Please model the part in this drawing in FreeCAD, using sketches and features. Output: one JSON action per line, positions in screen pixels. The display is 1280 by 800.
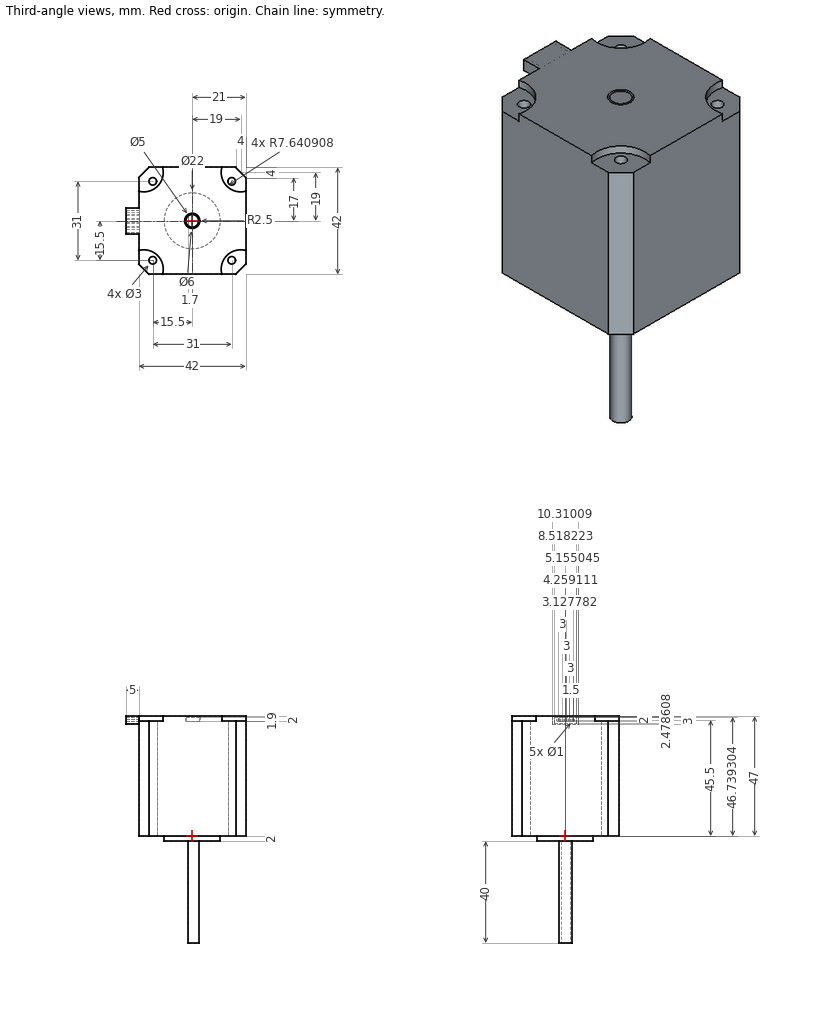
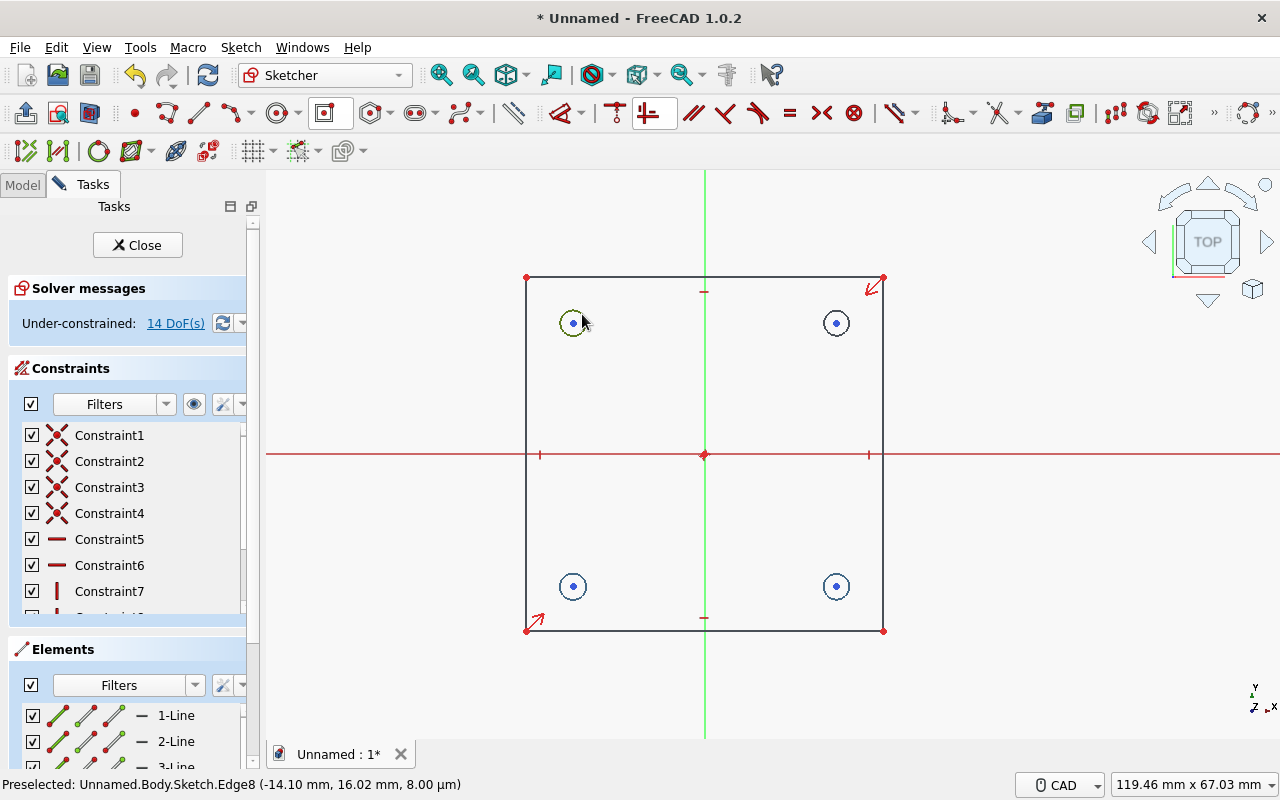
{"action": "left_click", "coordinate": [845, 314]}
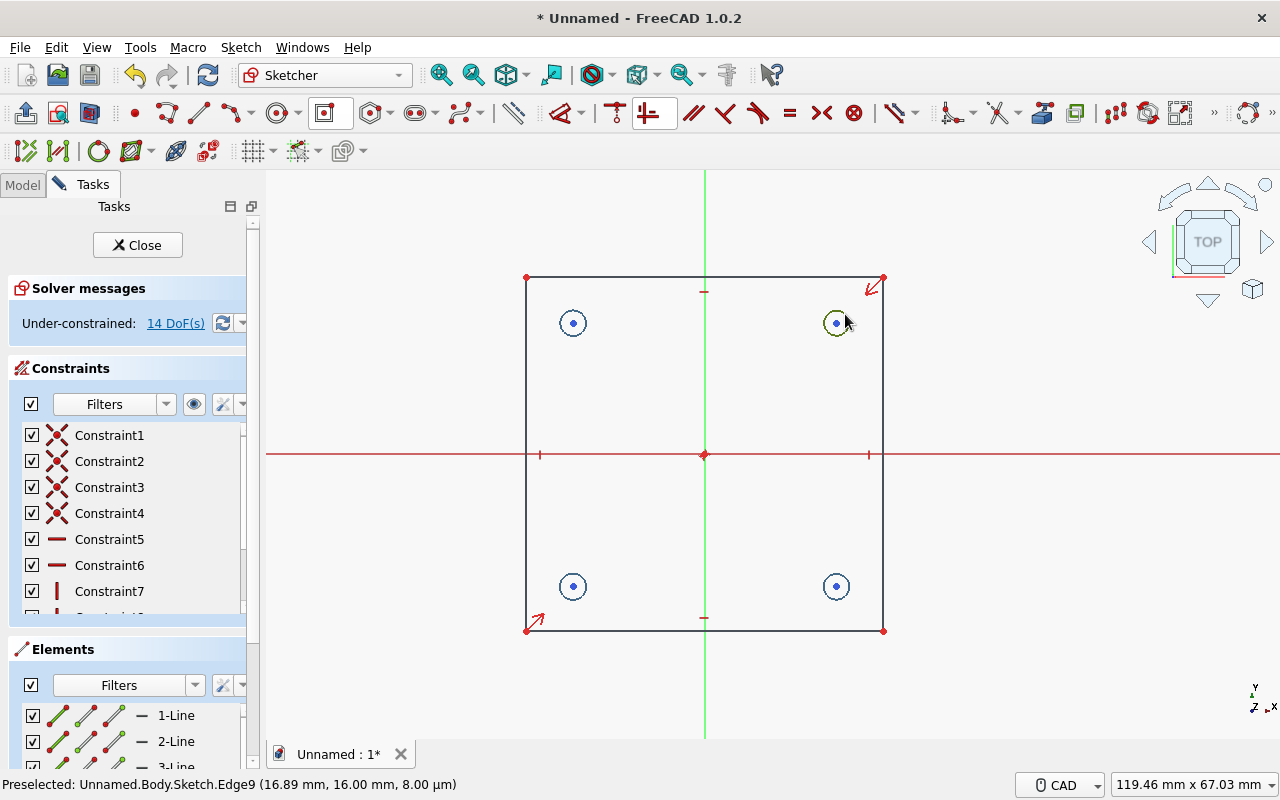
{"action": "left_click", "coordinate": [790, 114]}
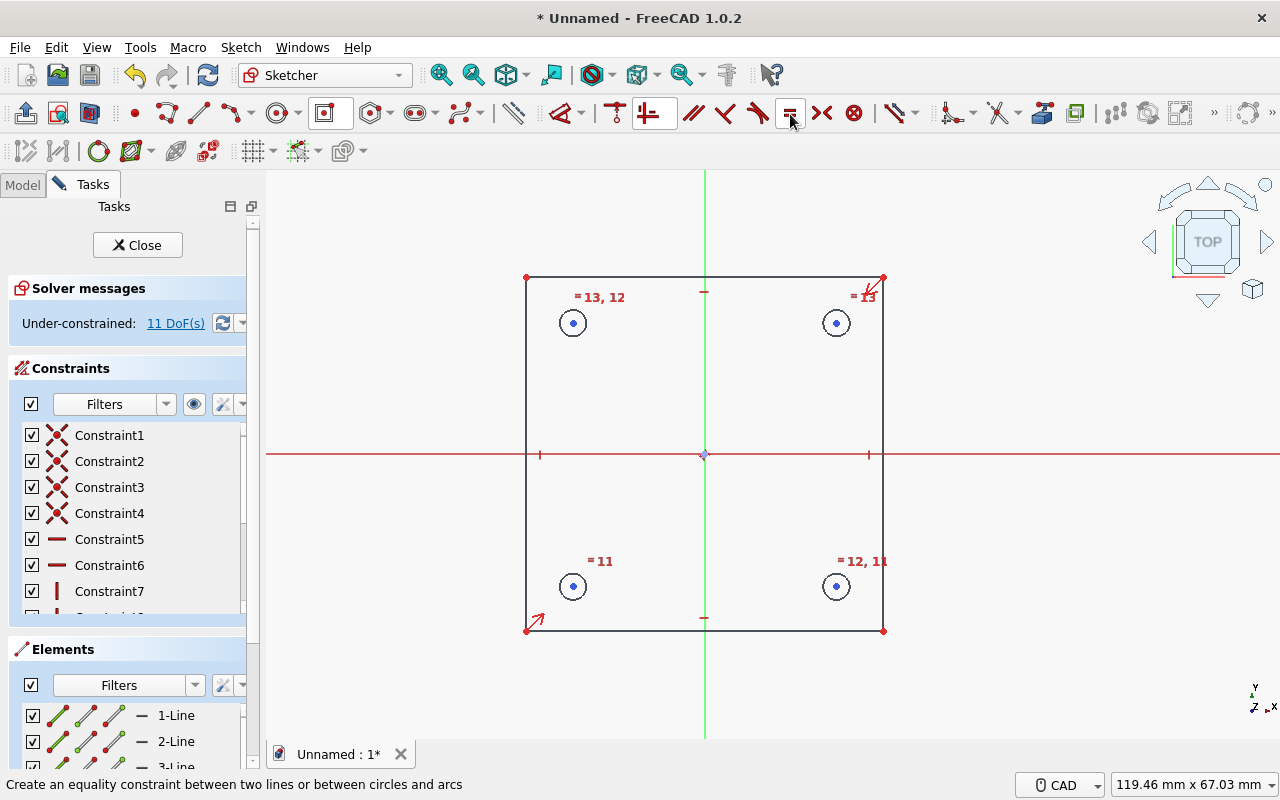
{"action": "left_click", "coordinate": [573, 587]}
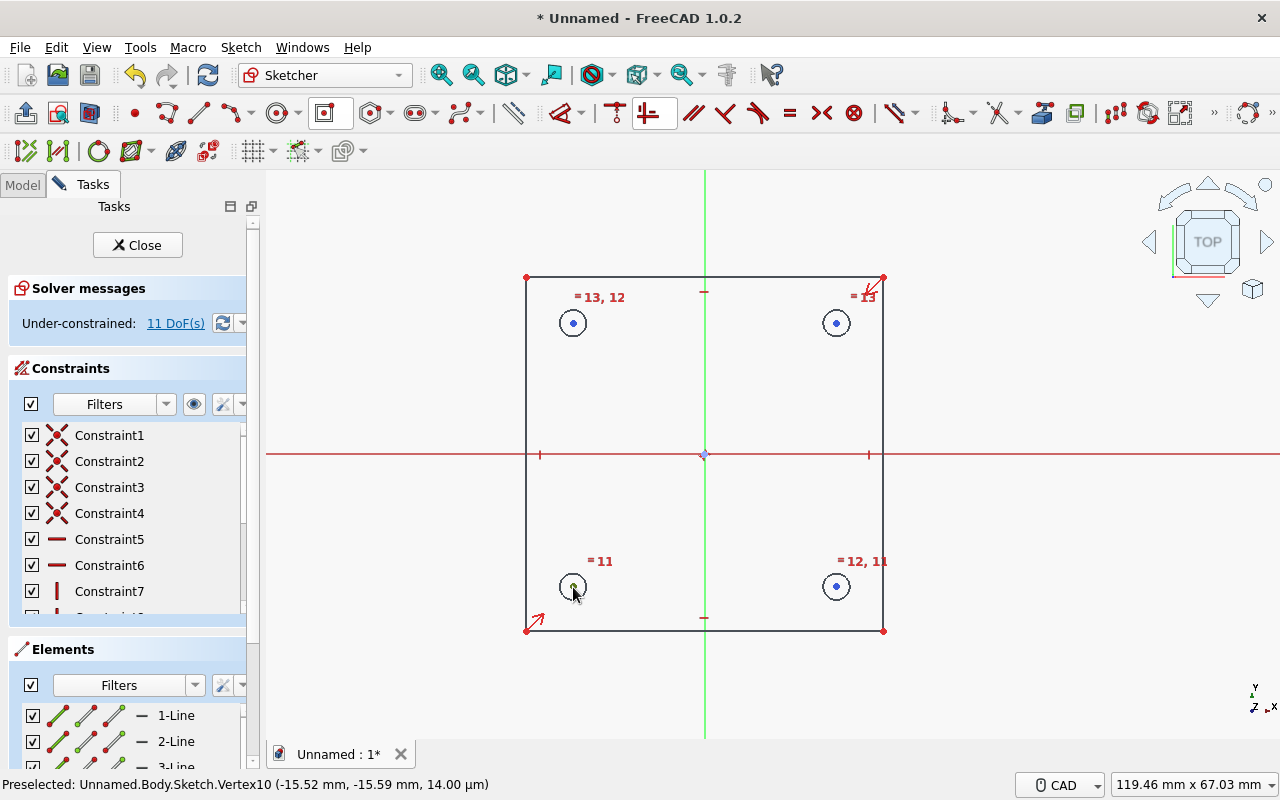
{"action": "left_click", "coordinate": [836, 587]}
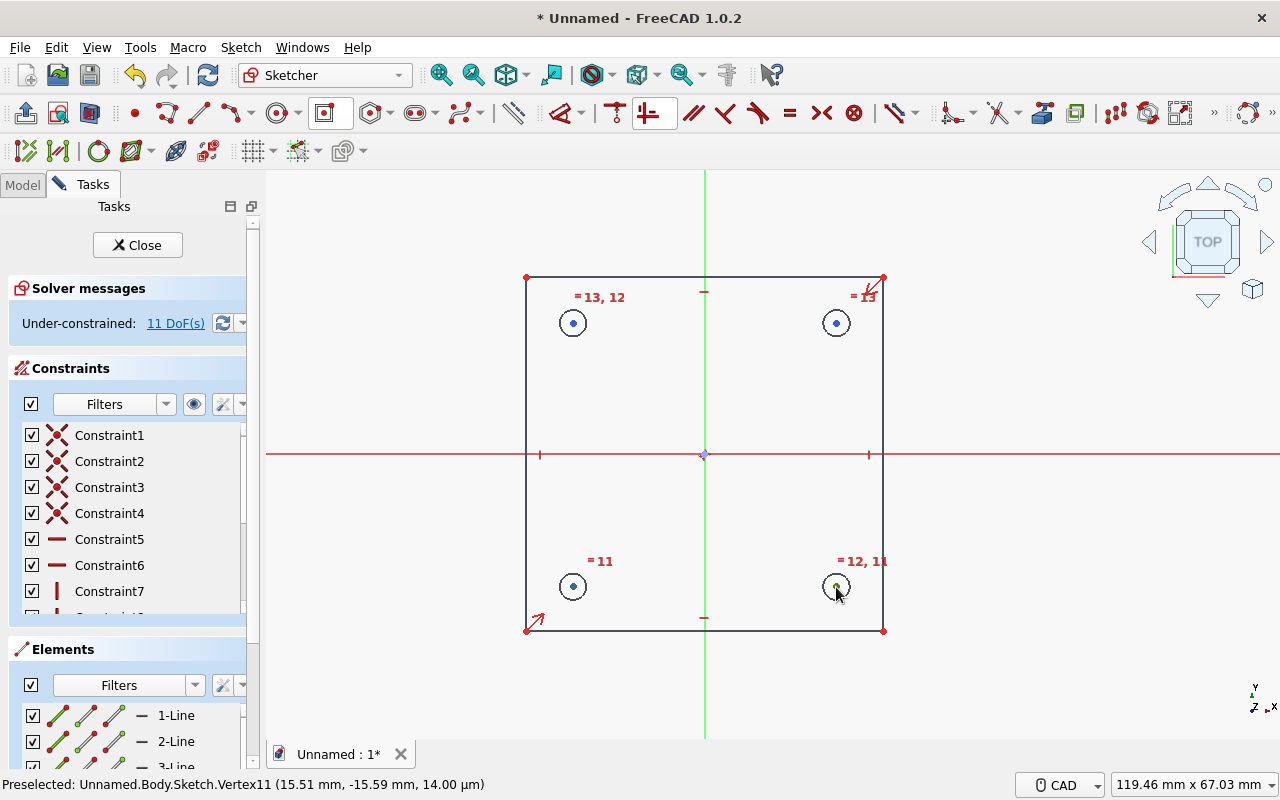
{"action": "left_click", "coordinate": [672, 114]}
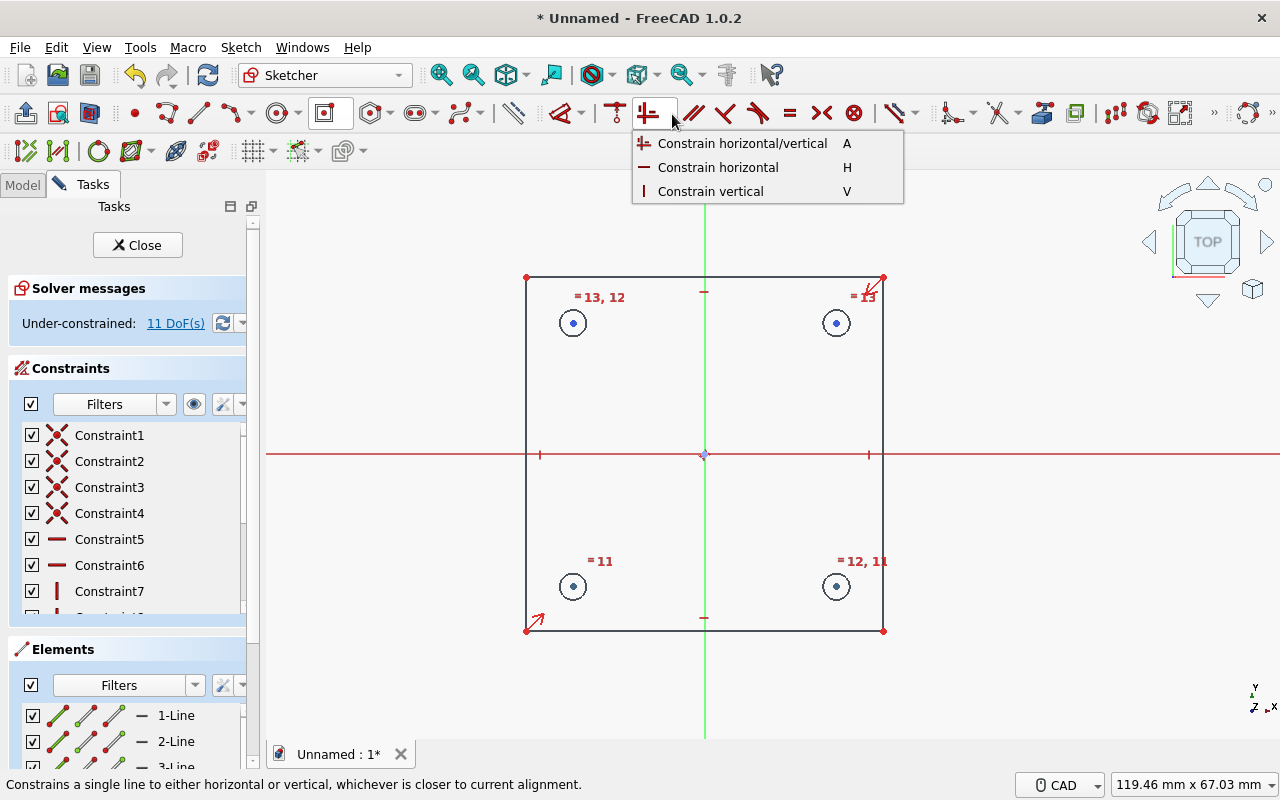
{"action": "left_click", "coordinate": [768, 167]}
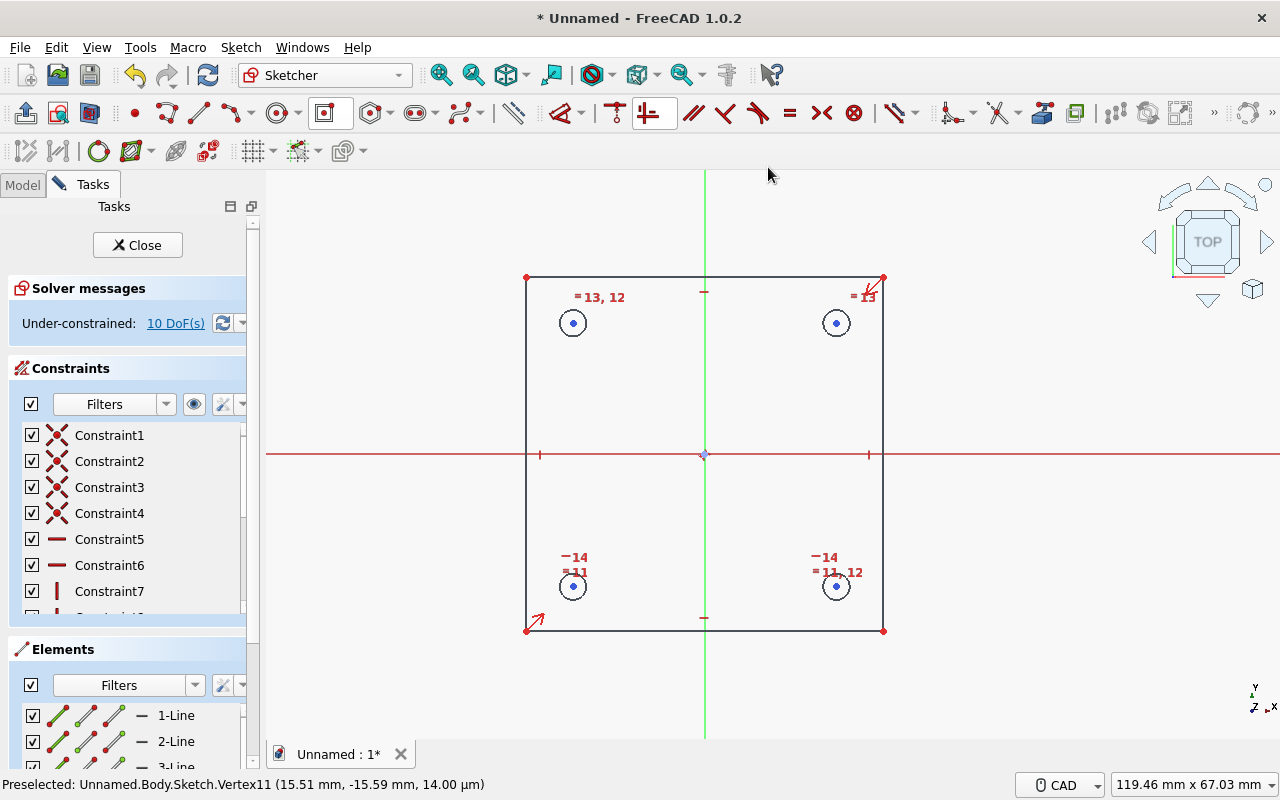
{"action": "left_click", "coordinate": [573, 587]}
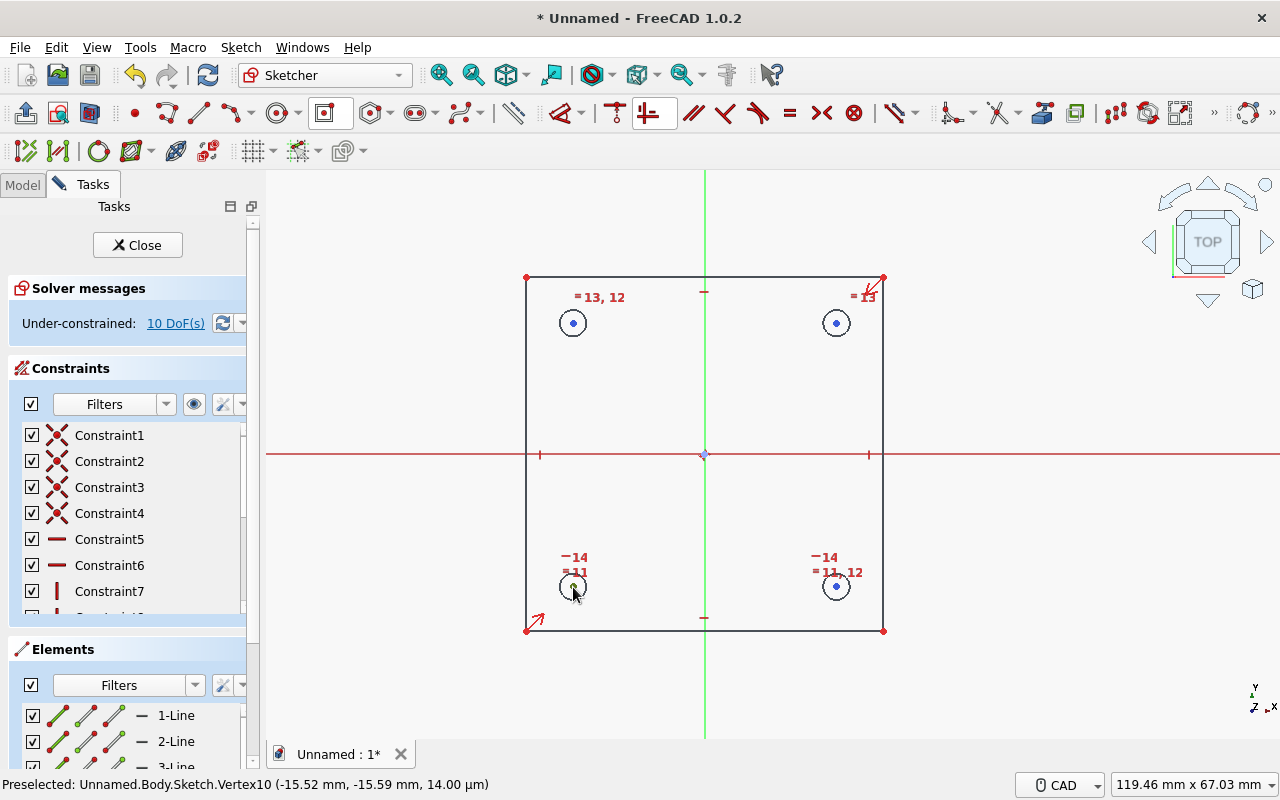
{"action": "left_click", "coordinate": [573, 323]}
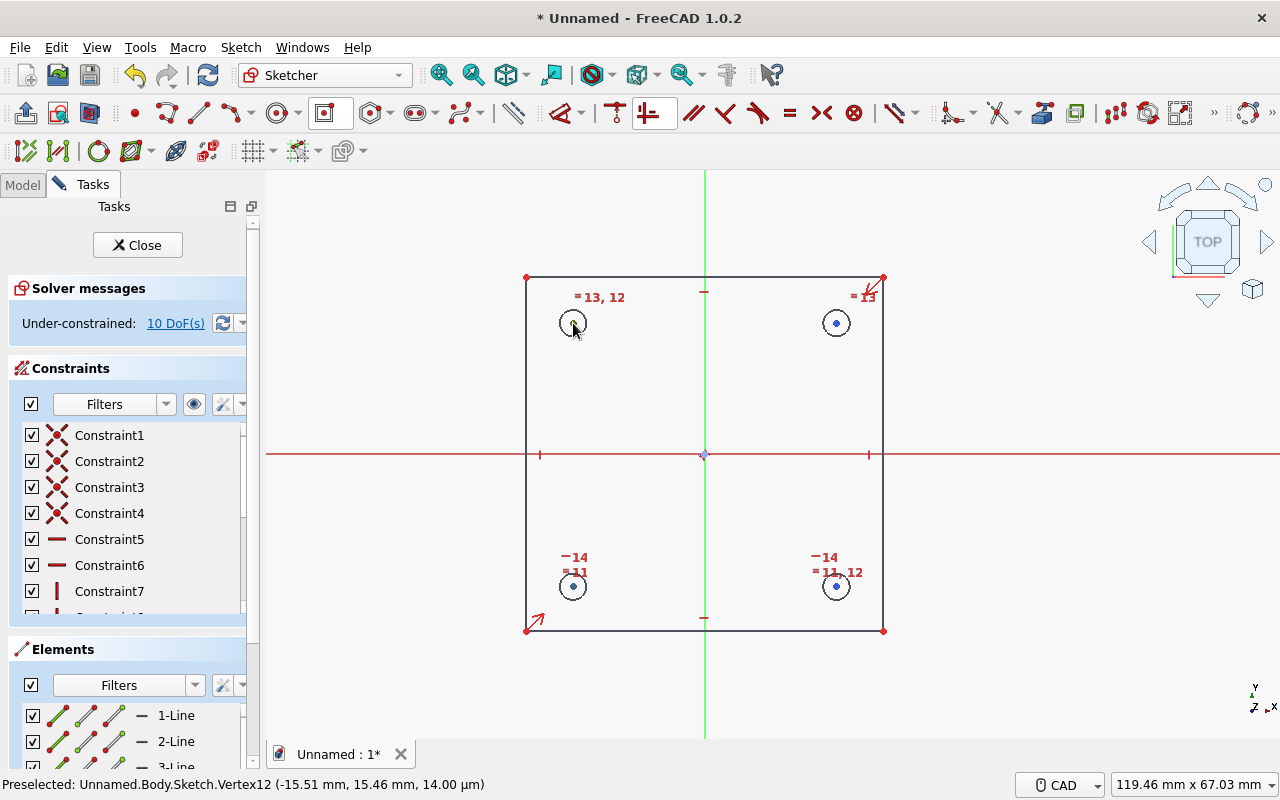
{"action": "key", "text": "v"}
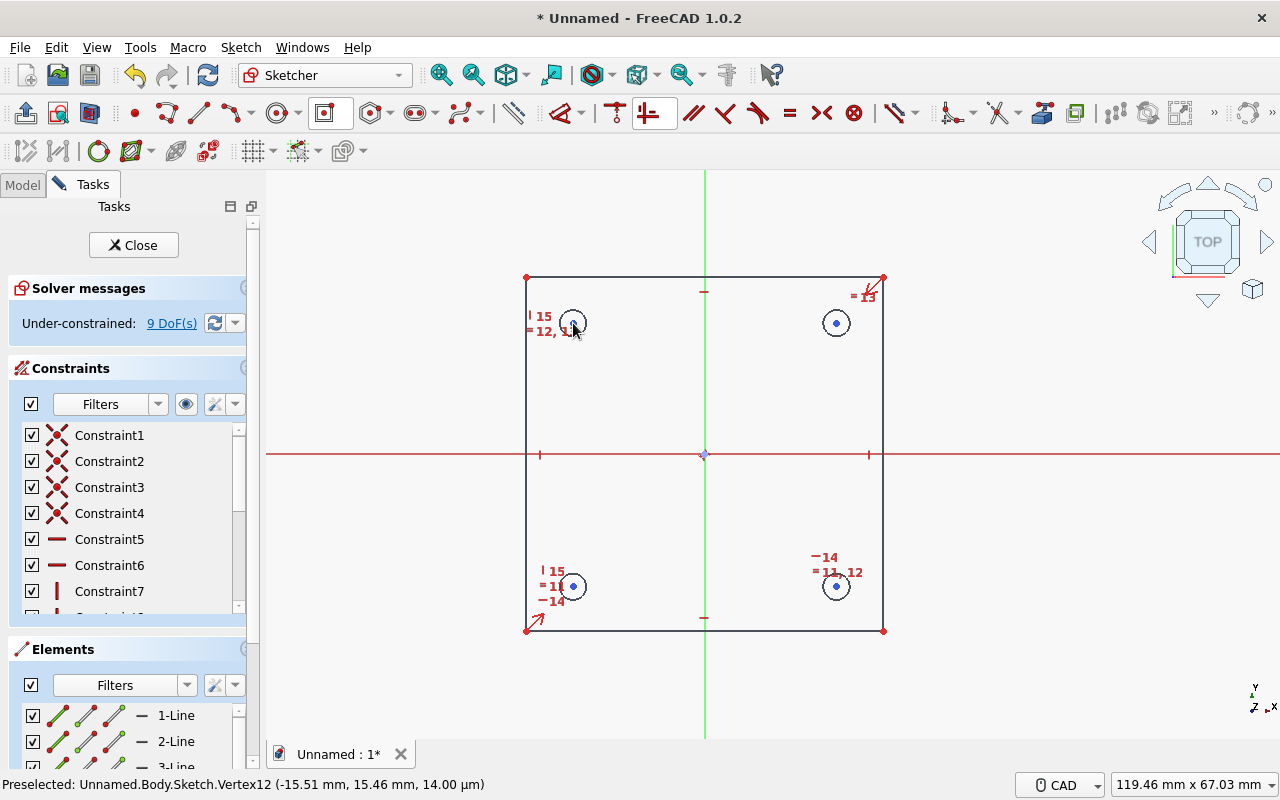
{"action": "left_click", "coordinate": [836, 587]}